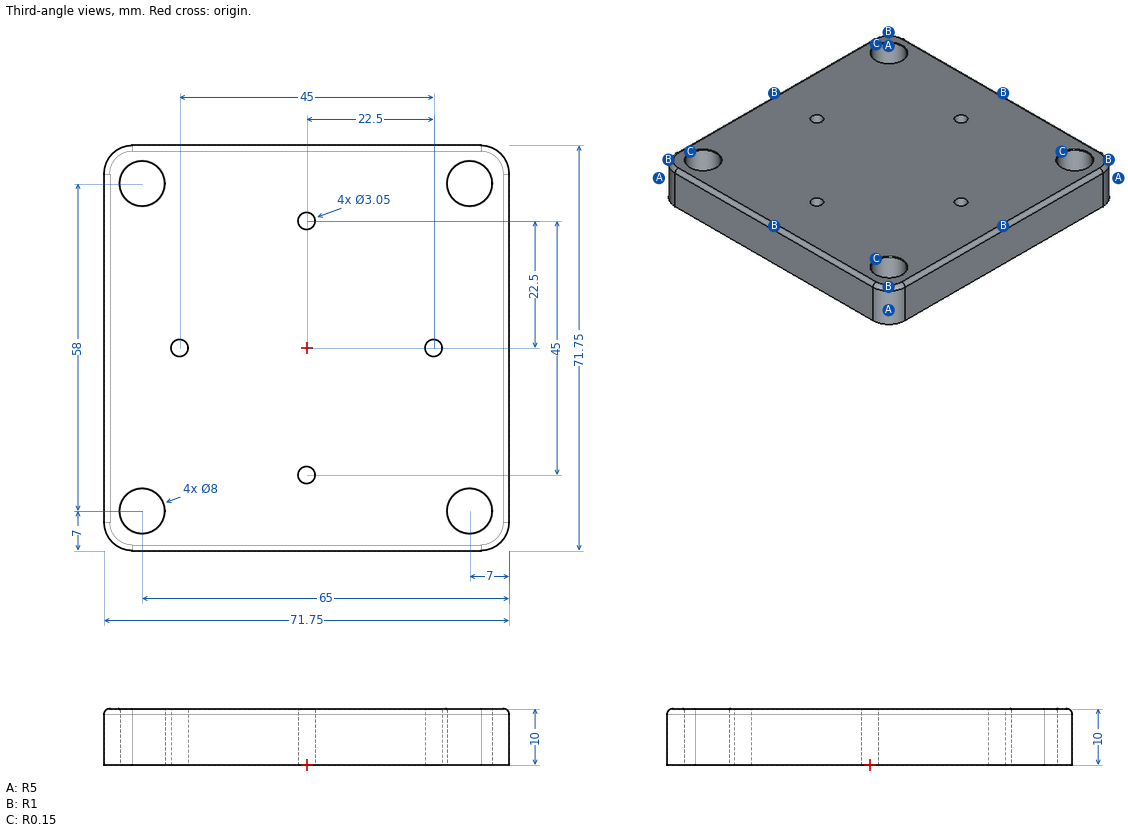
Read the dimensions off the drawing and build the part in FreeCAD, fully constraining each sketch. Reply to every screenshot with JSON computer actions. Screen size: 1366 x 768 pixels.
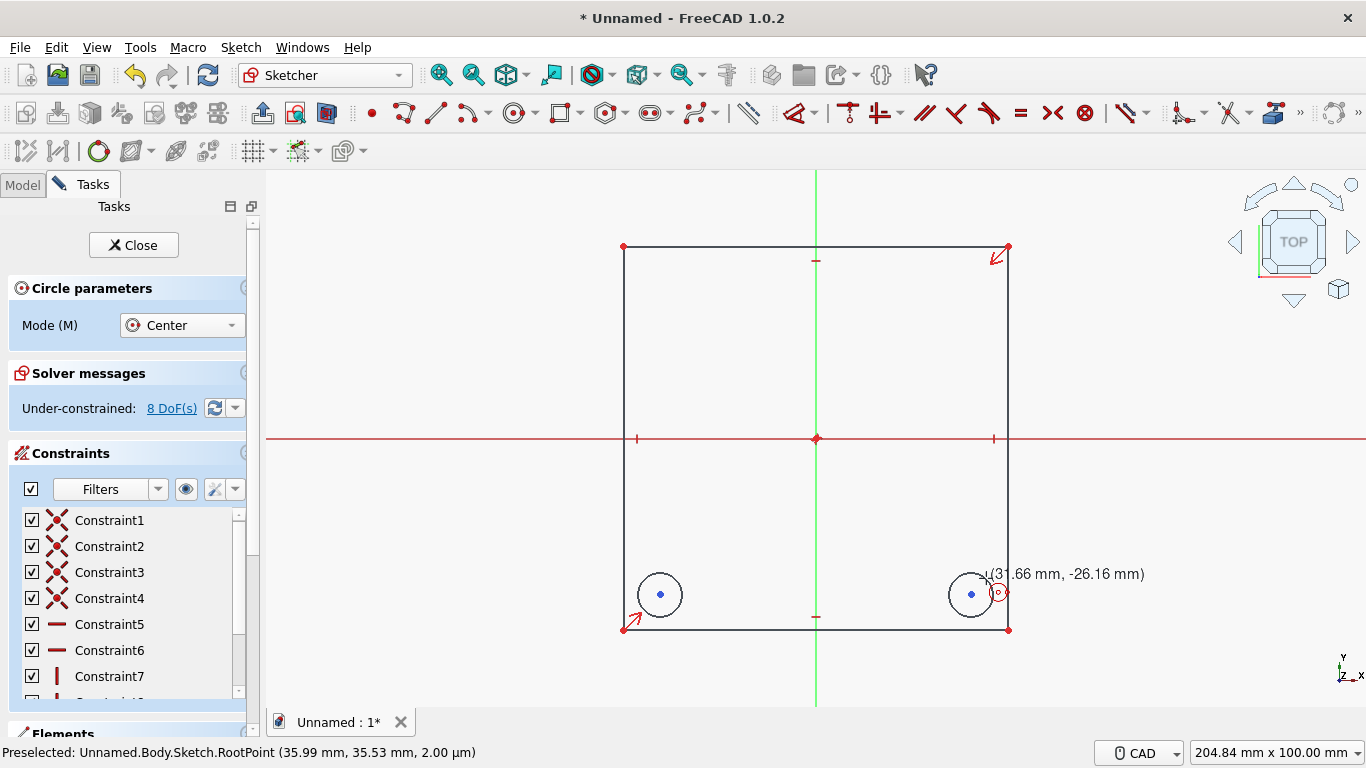
{"action": "left_click", "coordinate": [660, 282]}
{"action": "left_click", "coordinate": [675, 267]}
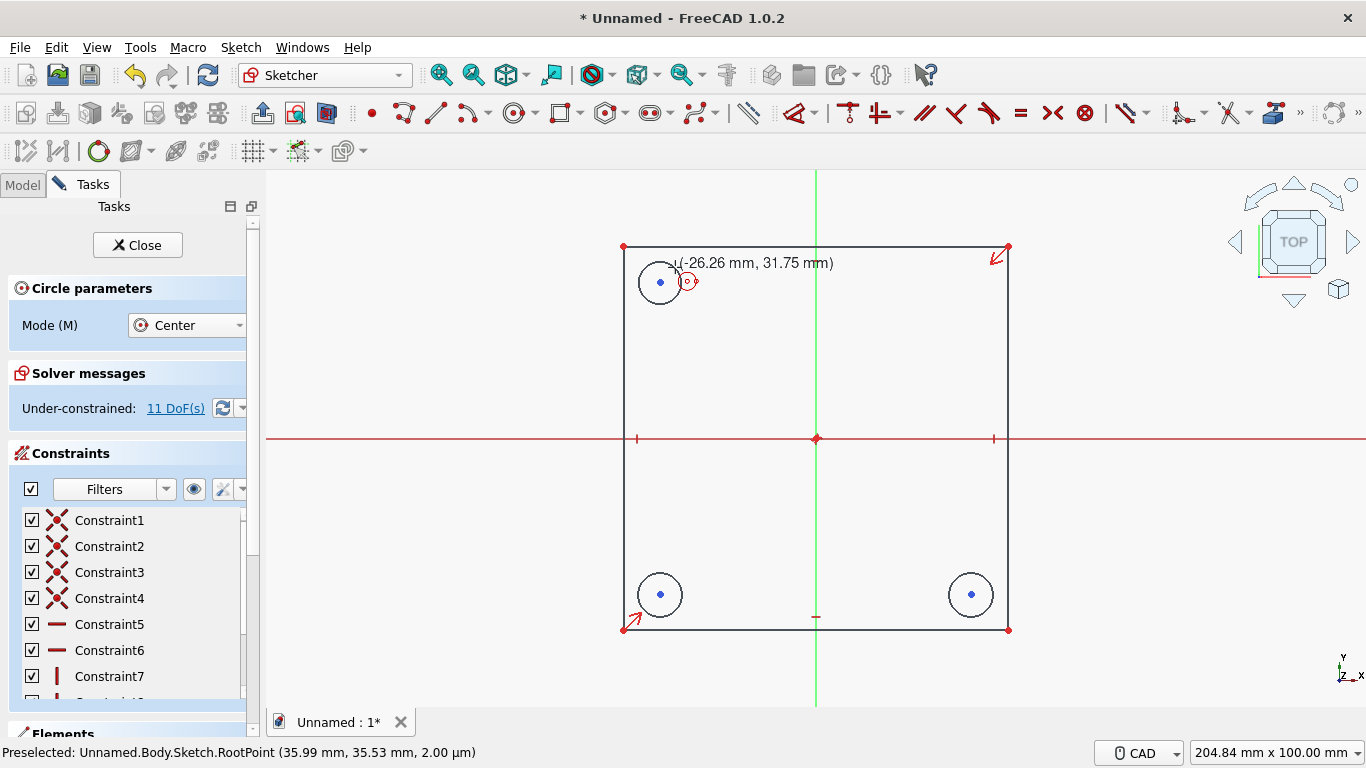
{"action": "left_click", "coordinate": [971, 282]}
{"action": "left_click", "coordinate": [986, 267]}
{"action": "key", "text": "Escape"}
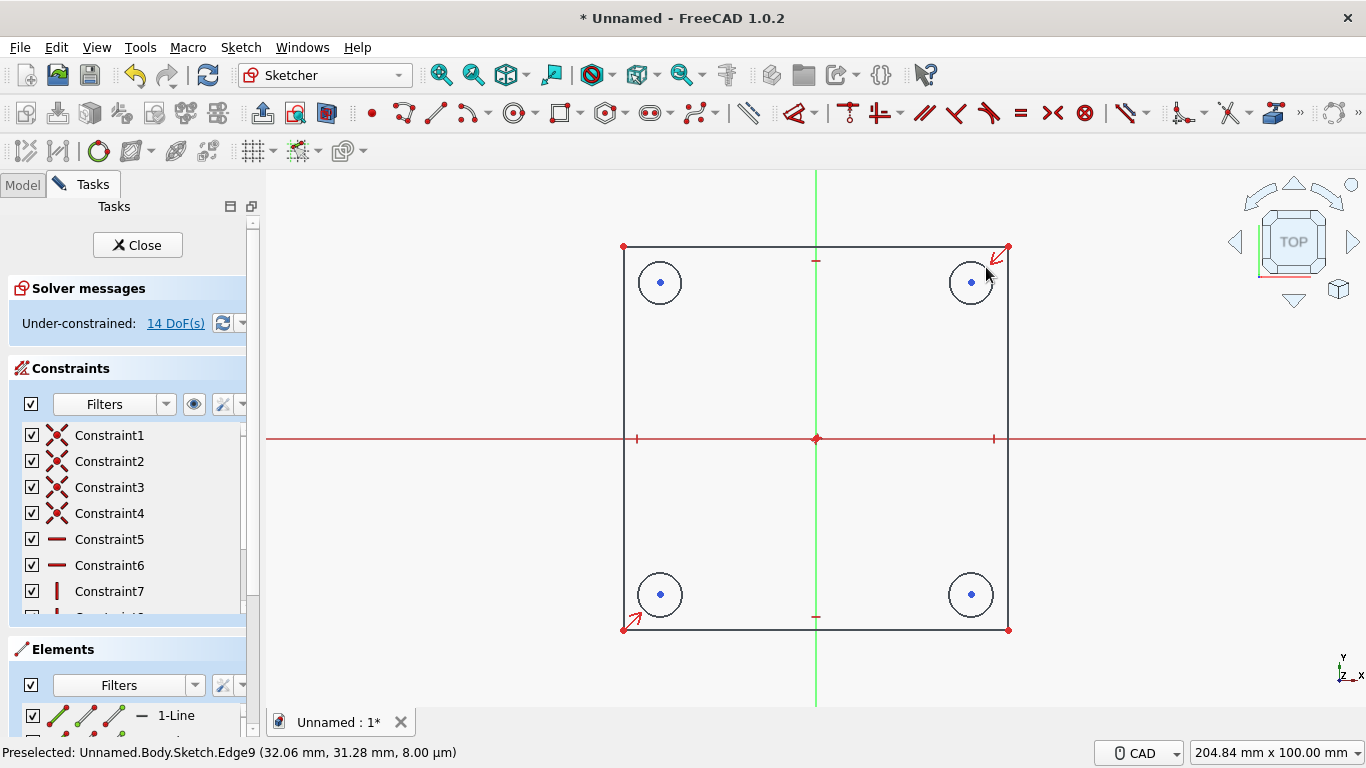
{"action": "left_click", "coordinate": [675, 579]}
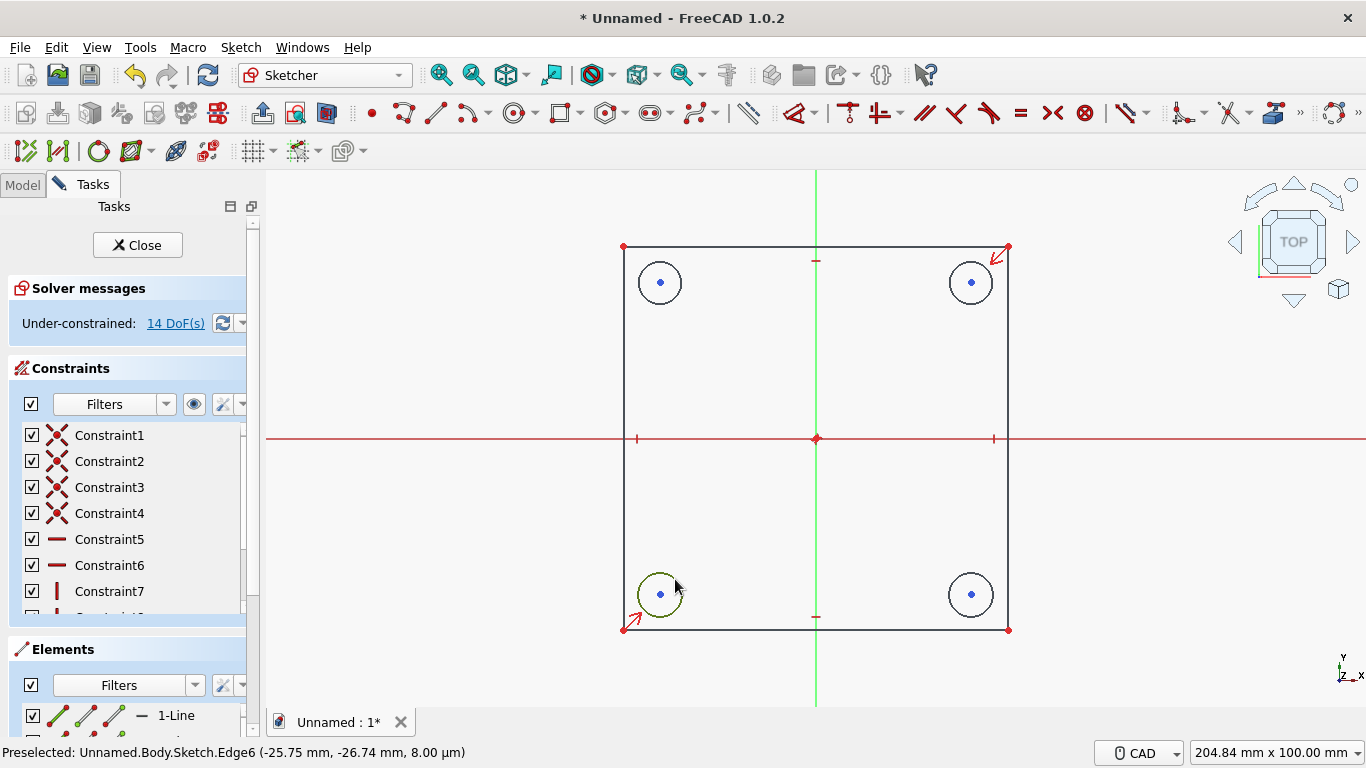
{"action": "left_click", "coordinate": [986, 579]}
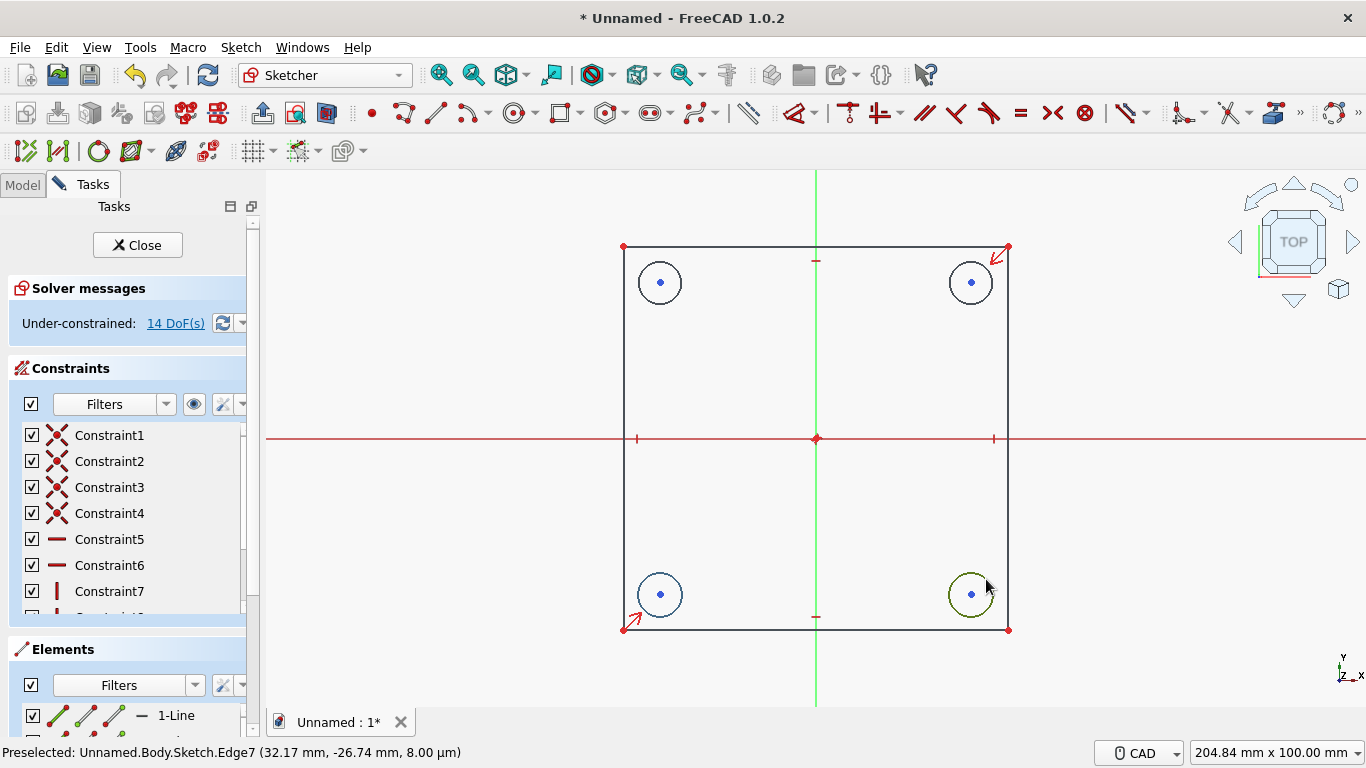
{"action": "left_click", "coordinate": [675, 268]}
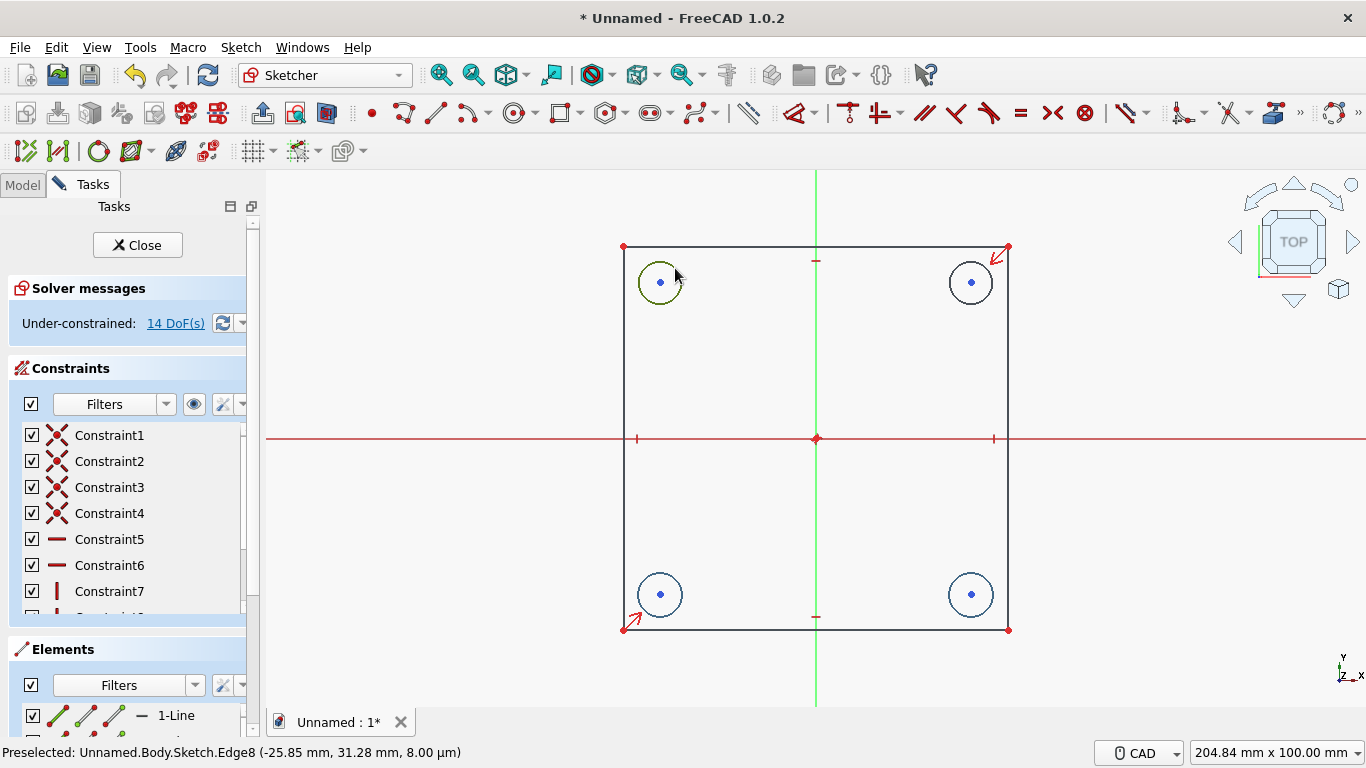
{"action": "left_click", "coordinate": [986, 268]}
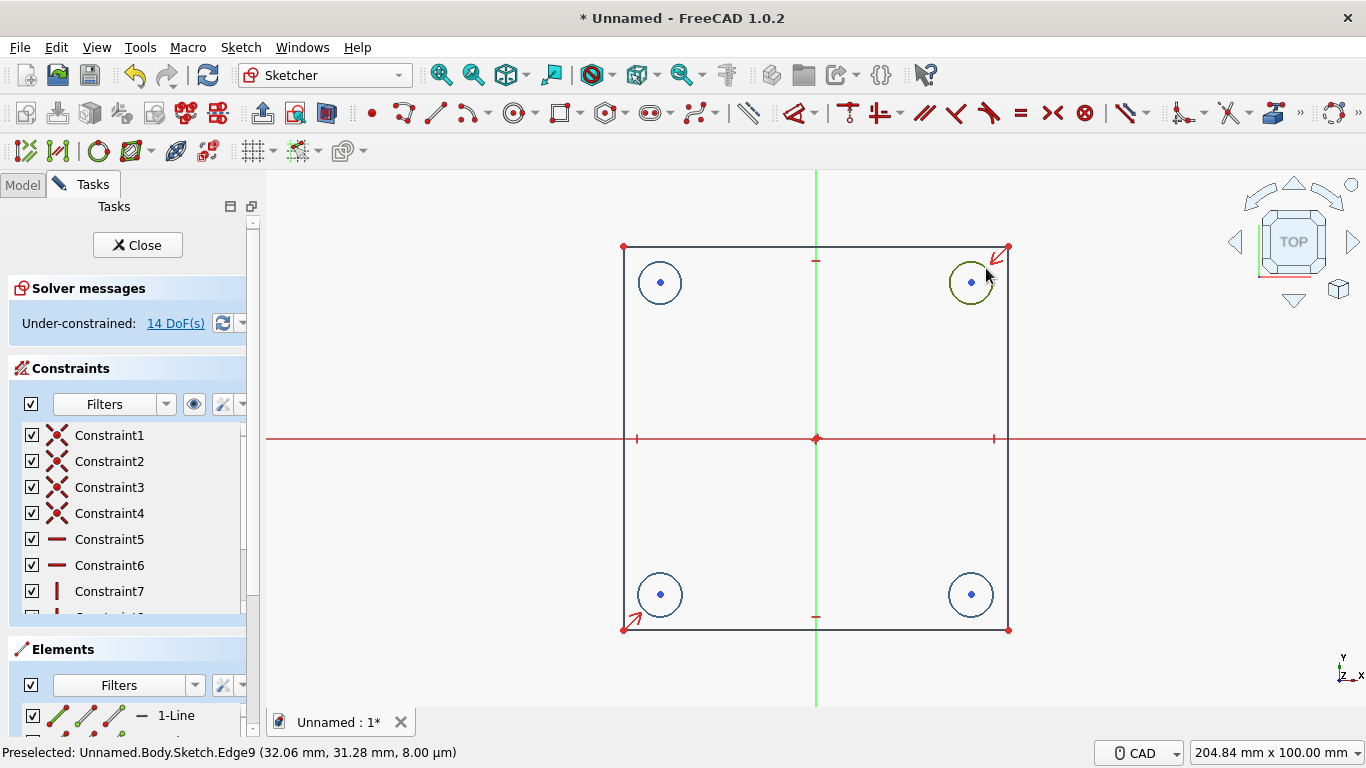
{"action": "left_click", "coordinate": [1022, 114]}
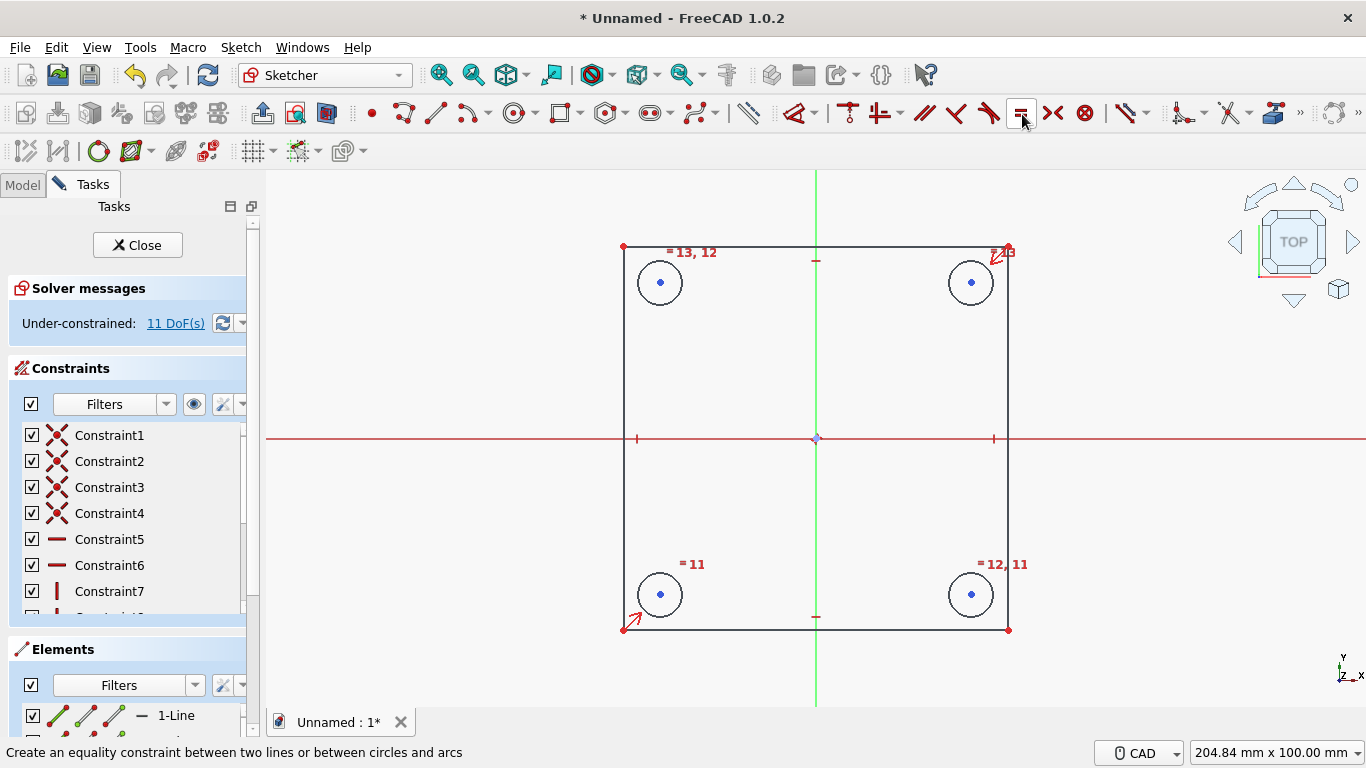
{"action": "left_click", "coordinate": [794, 114]}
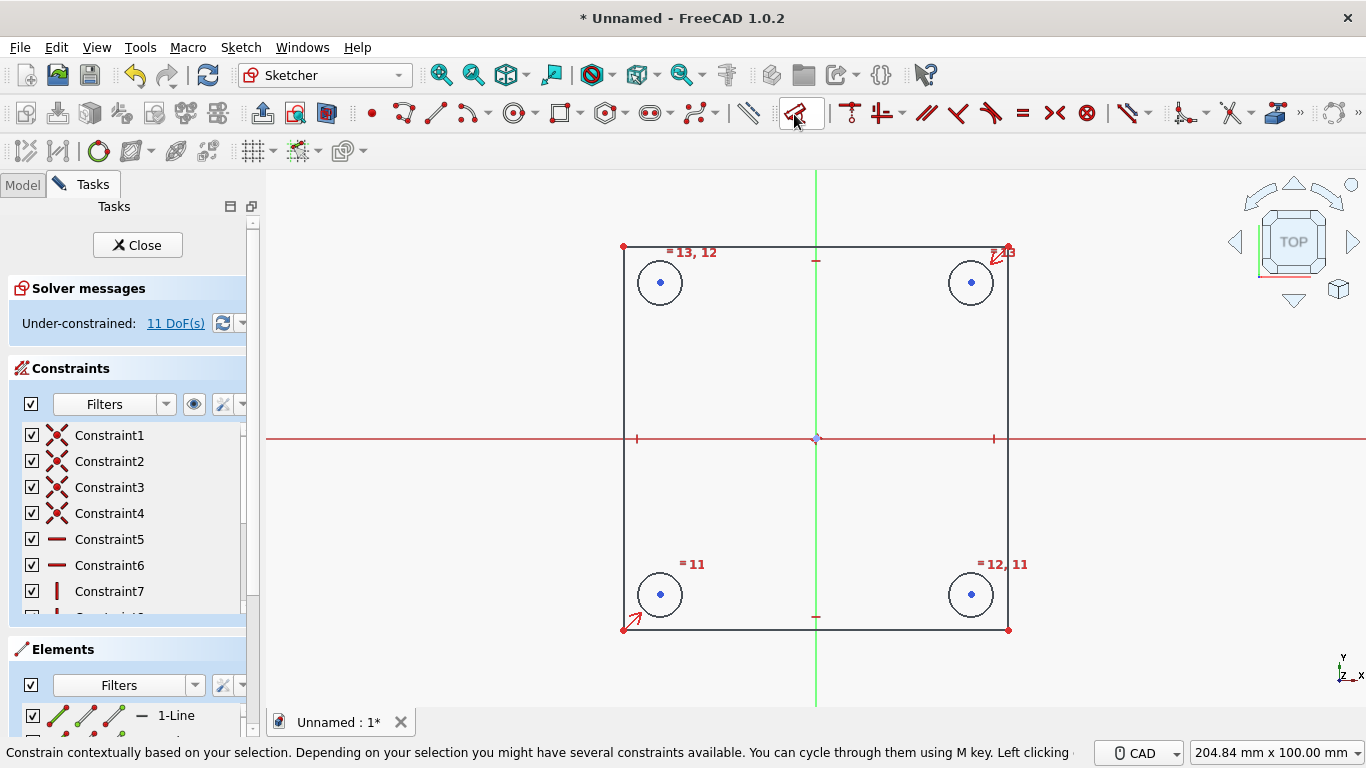
{"action": "left_click", "coordinate": [675, 579]}
{"action": "left_click", "coordinate": [697, 556]}